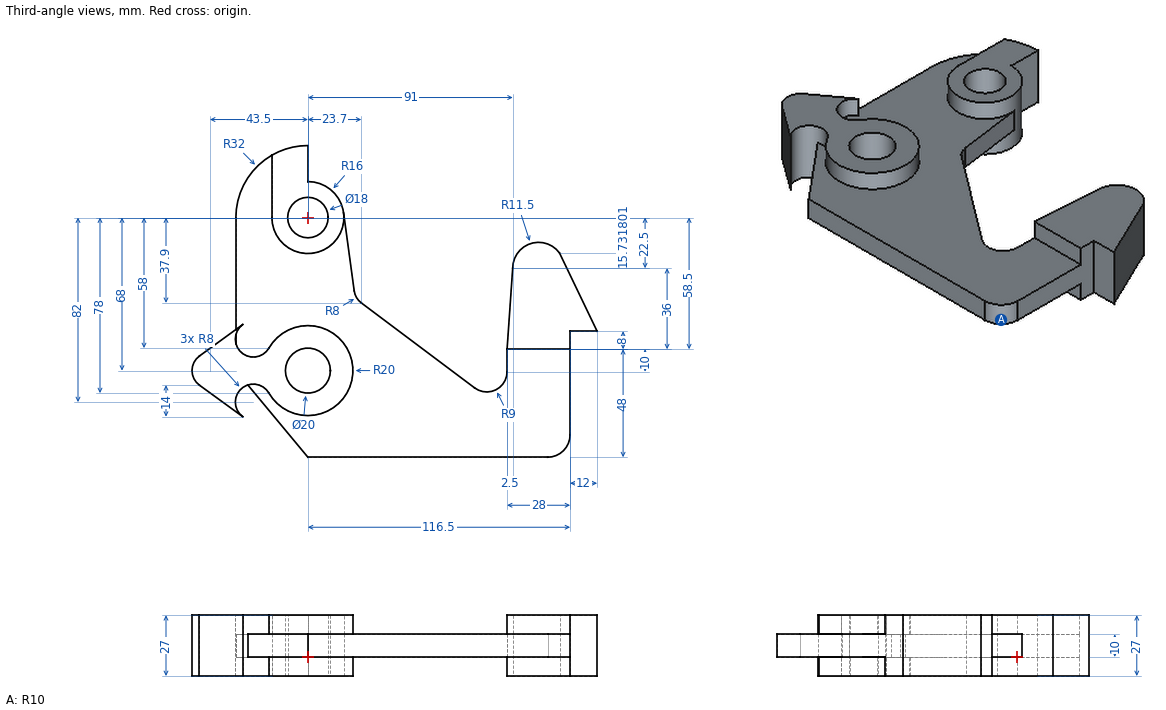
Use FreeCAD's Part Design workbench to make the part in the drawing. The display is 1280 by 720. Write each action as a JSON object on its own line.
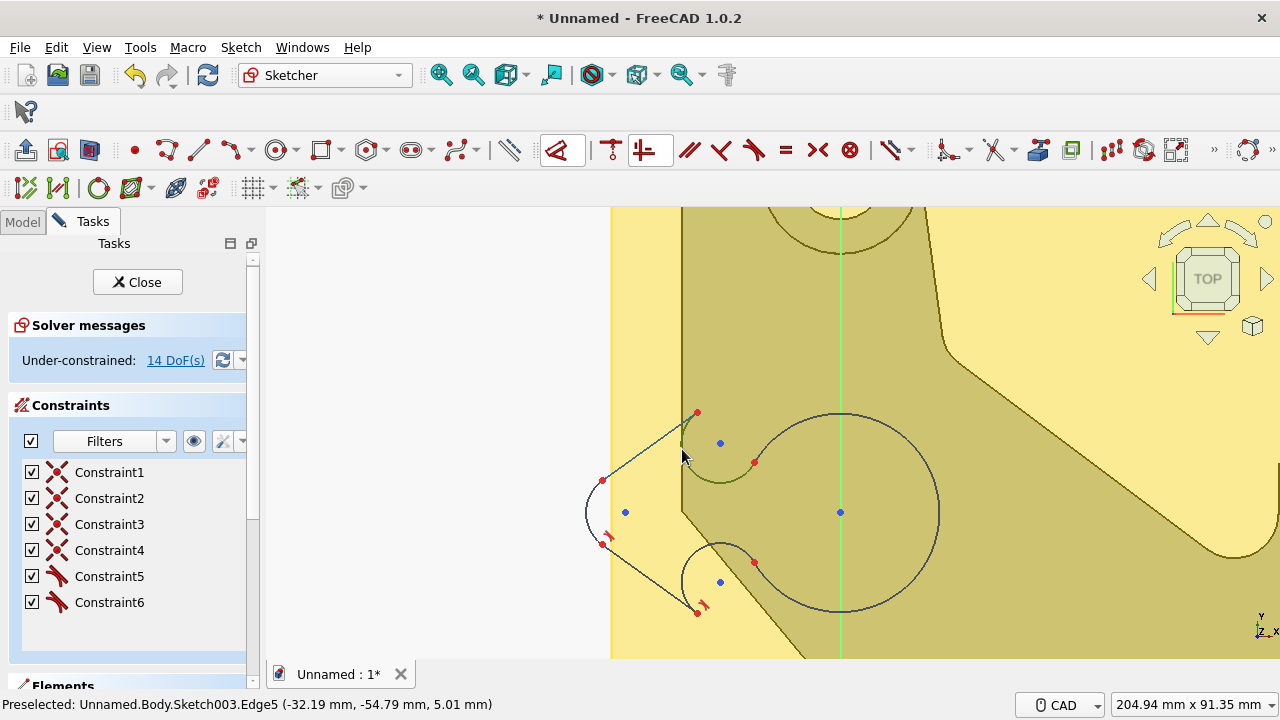
{"action": "key", "text": "t"}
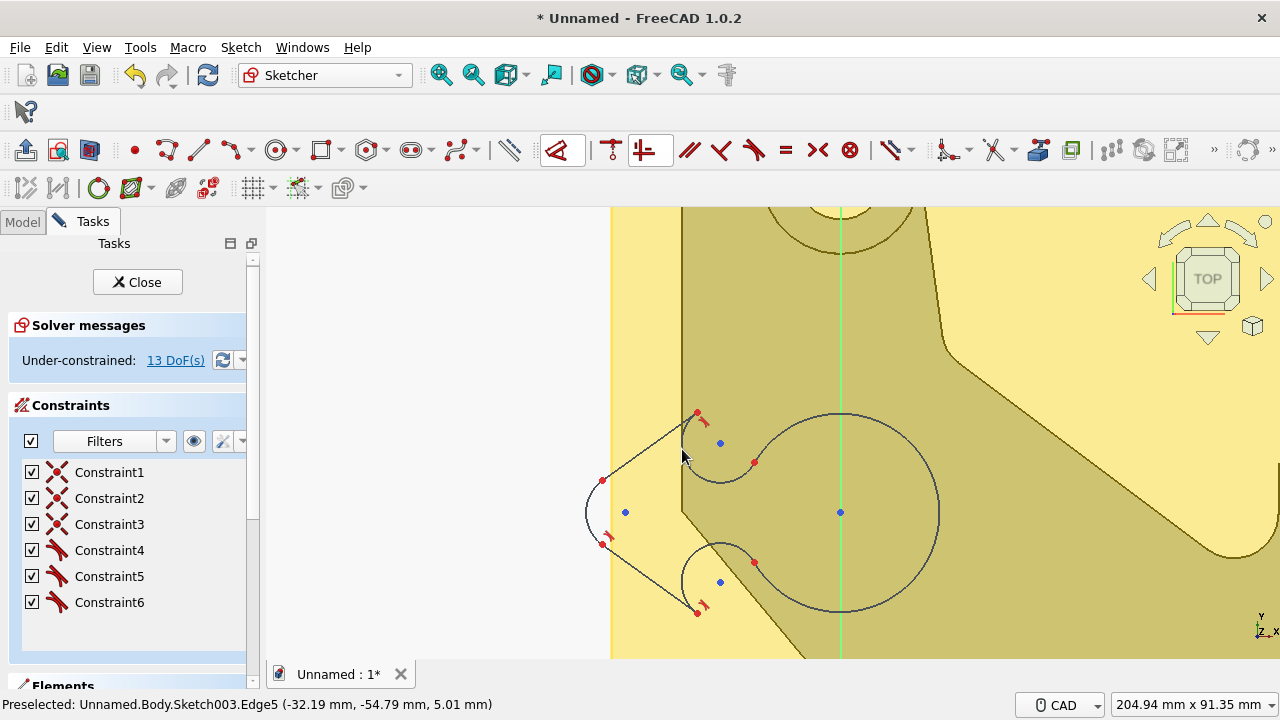
{"action": "left_click", "coordinate": [669, 433]}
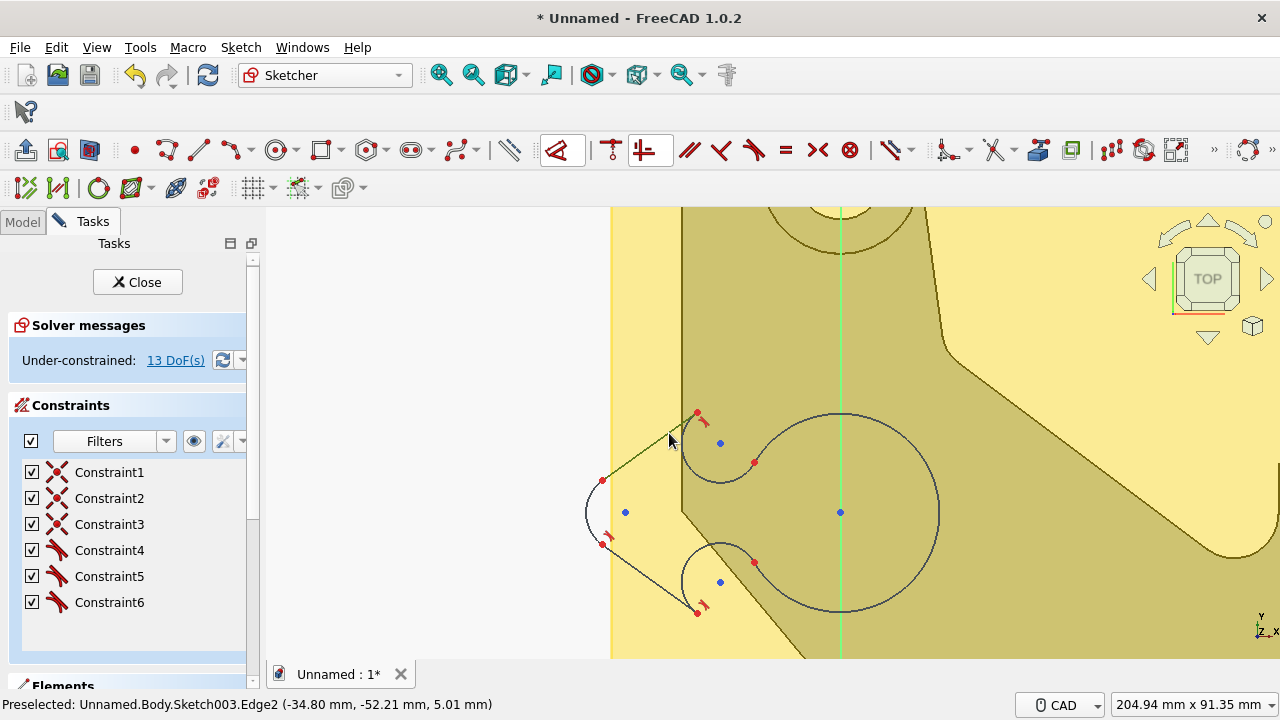
{"action": "left_click", "coordinate": [589, 498]}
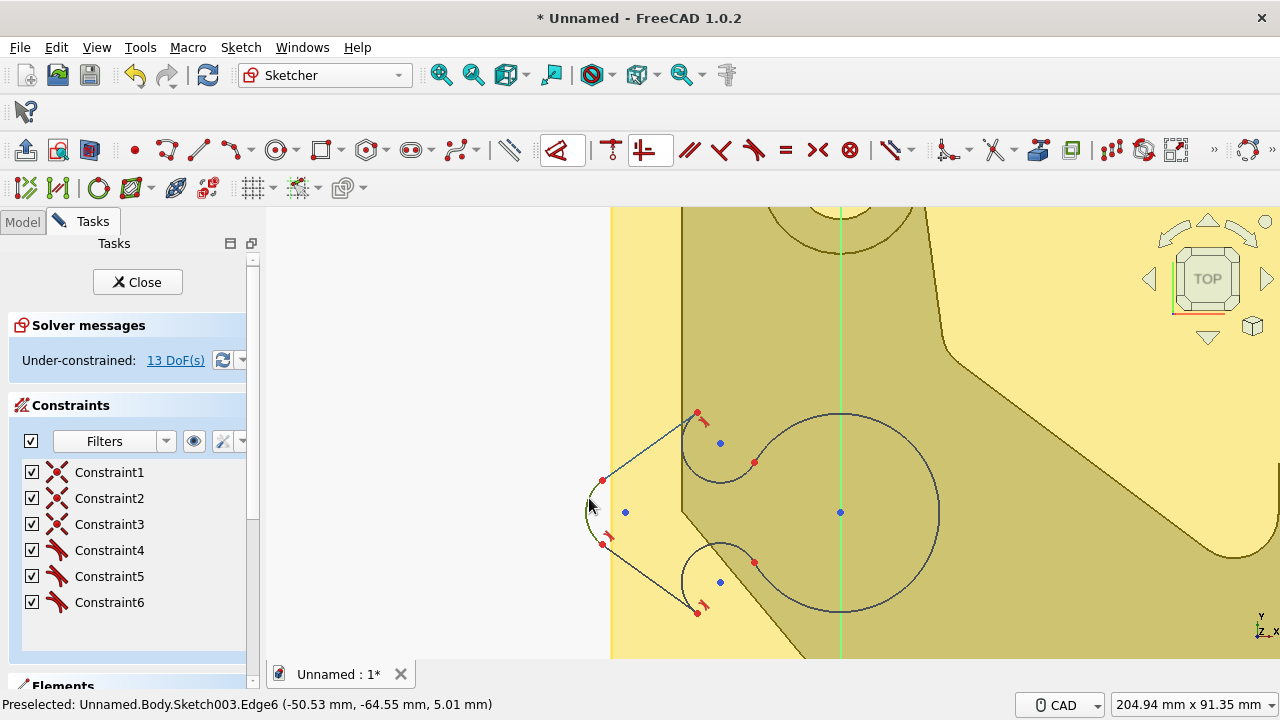
{"action": "left_click", "coordinate": [754, 150]}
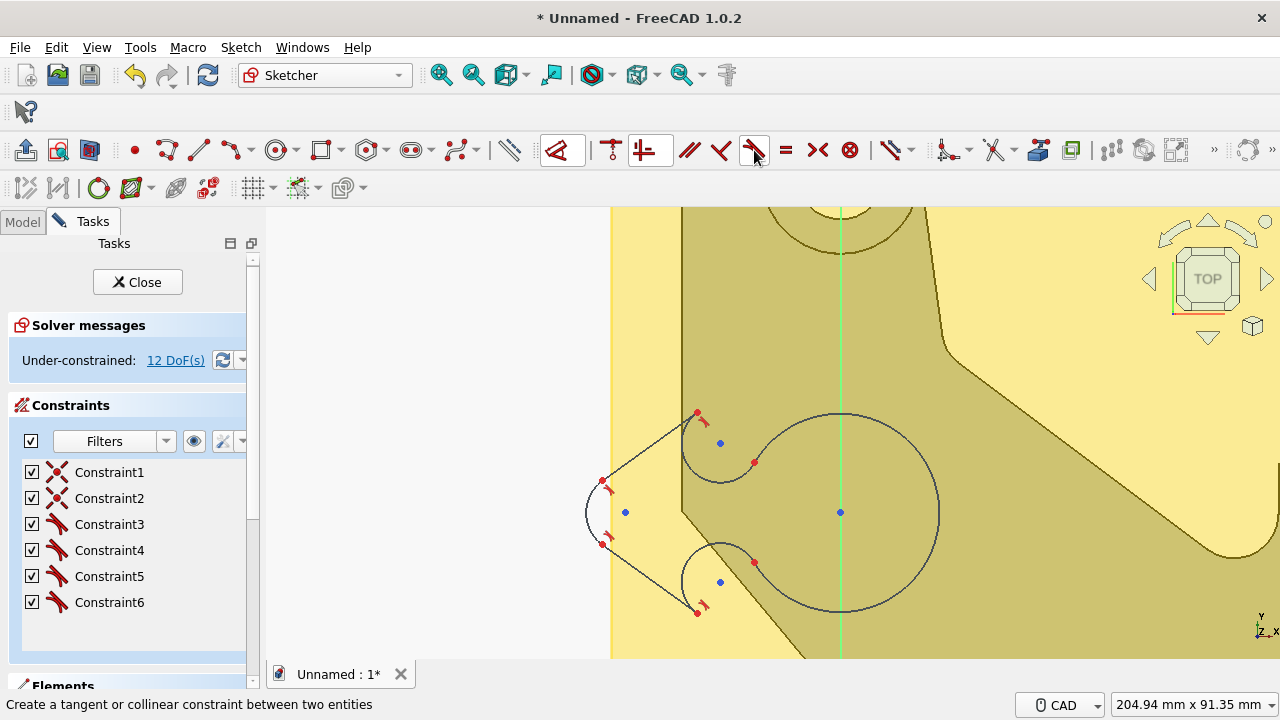
{"action": "left_click", "coordinate": [720, 543]}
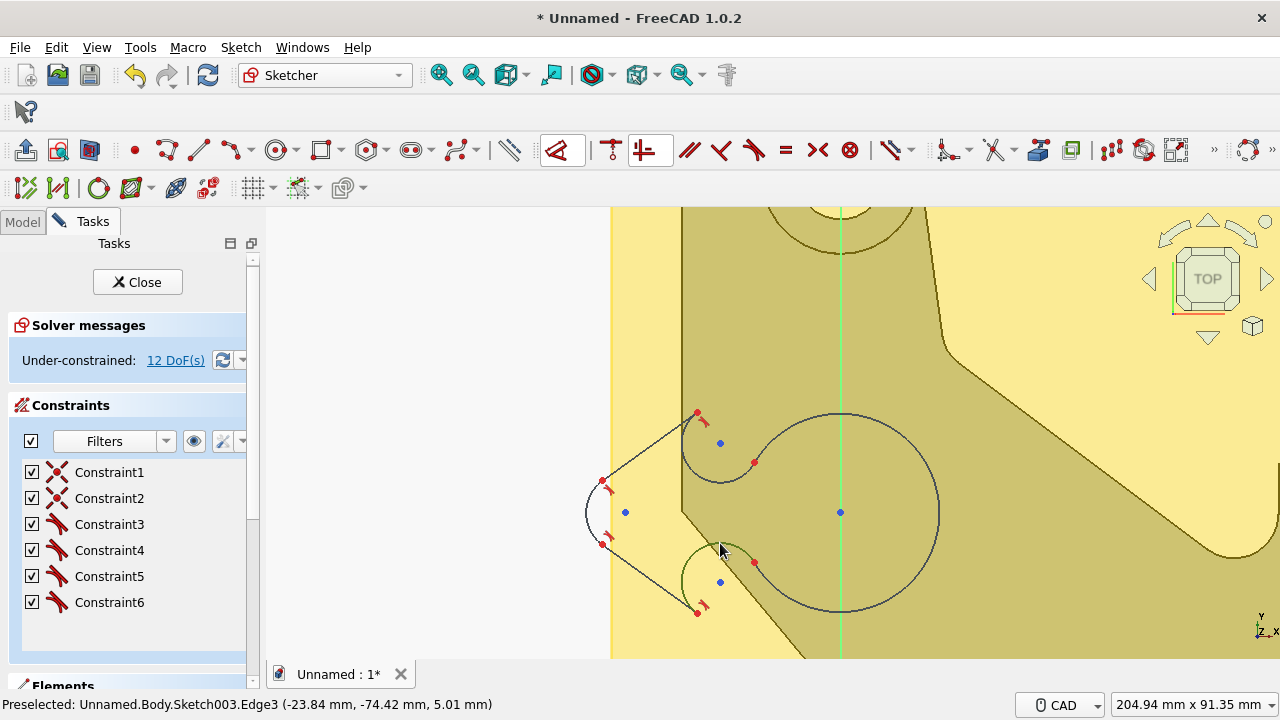
{"action": "left_click", "coordinate": [890, 599]}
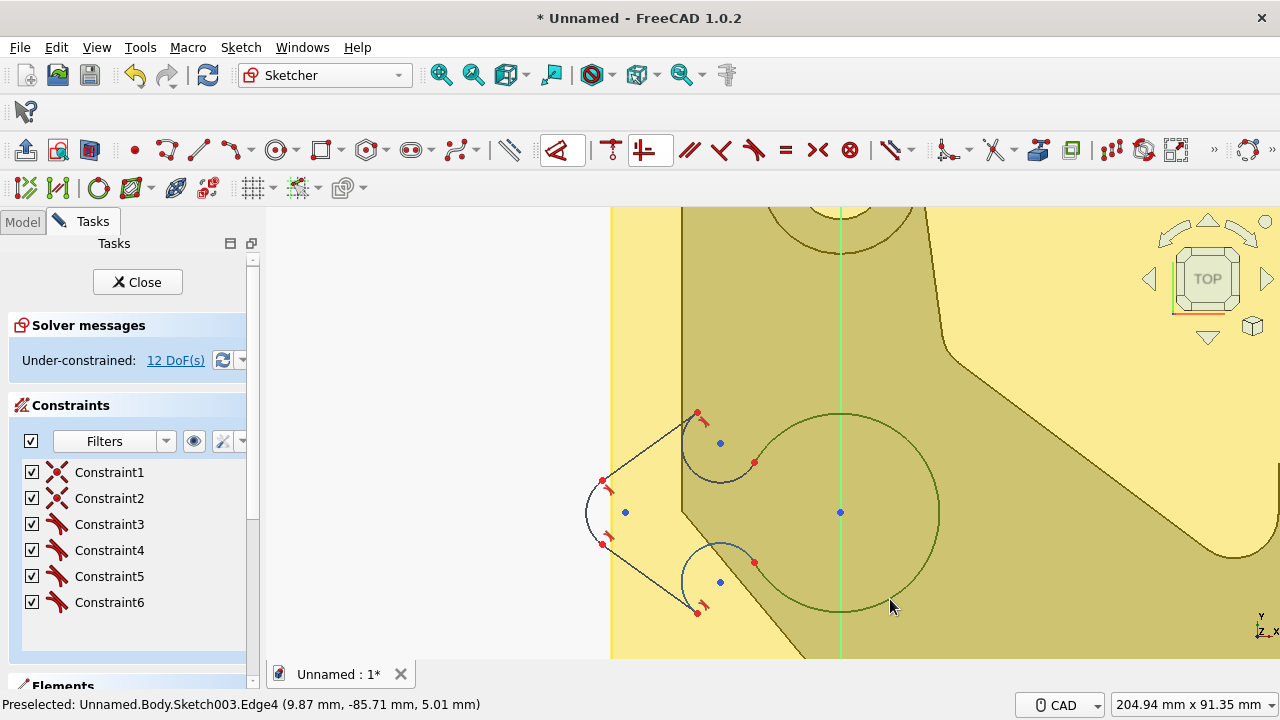
{"action": "key", "text": "t"}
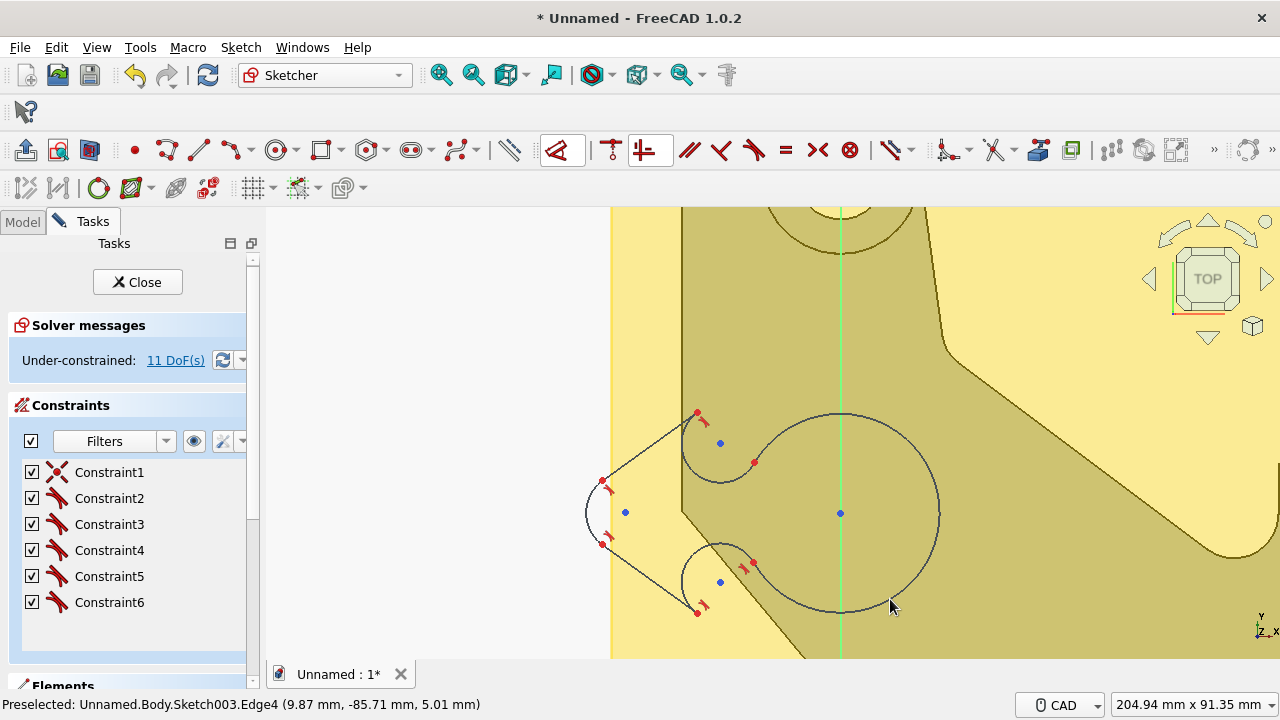
{"action": "left_click", "coordinate": [890, 600]}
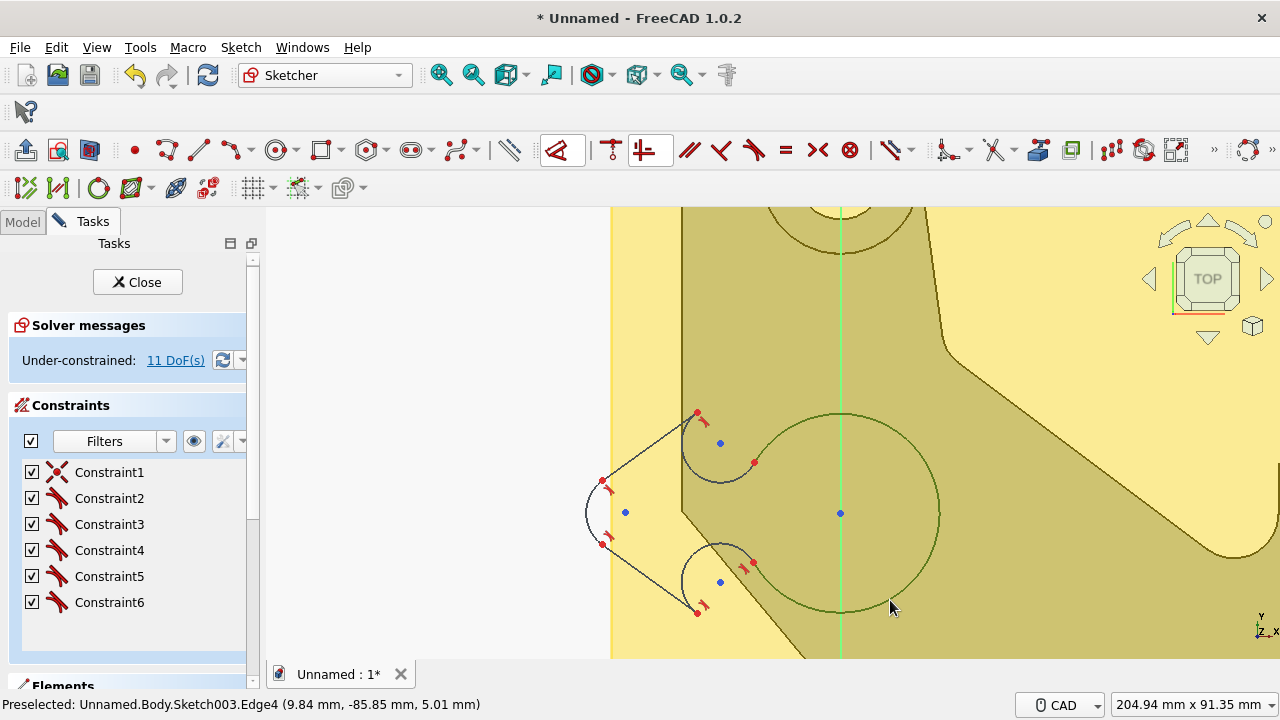
{"action": "left_click", "coordinate": [682, 449]}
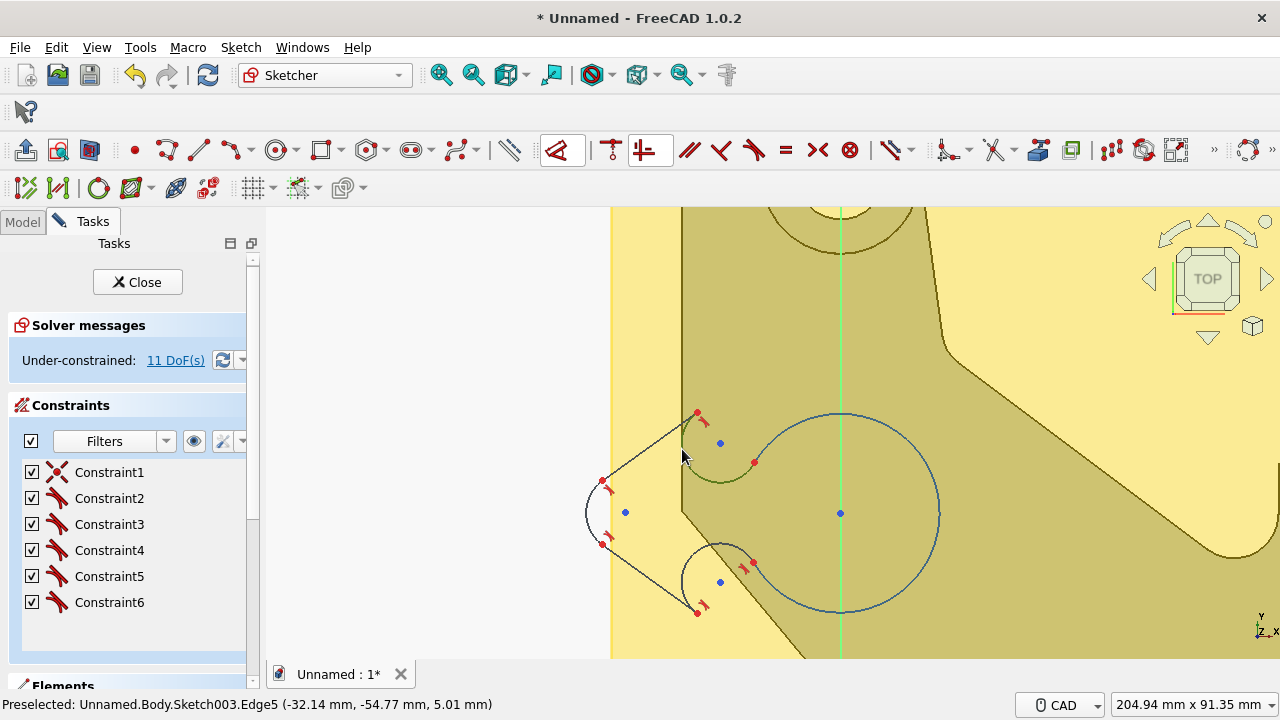
{"action": "key", "text": "t"}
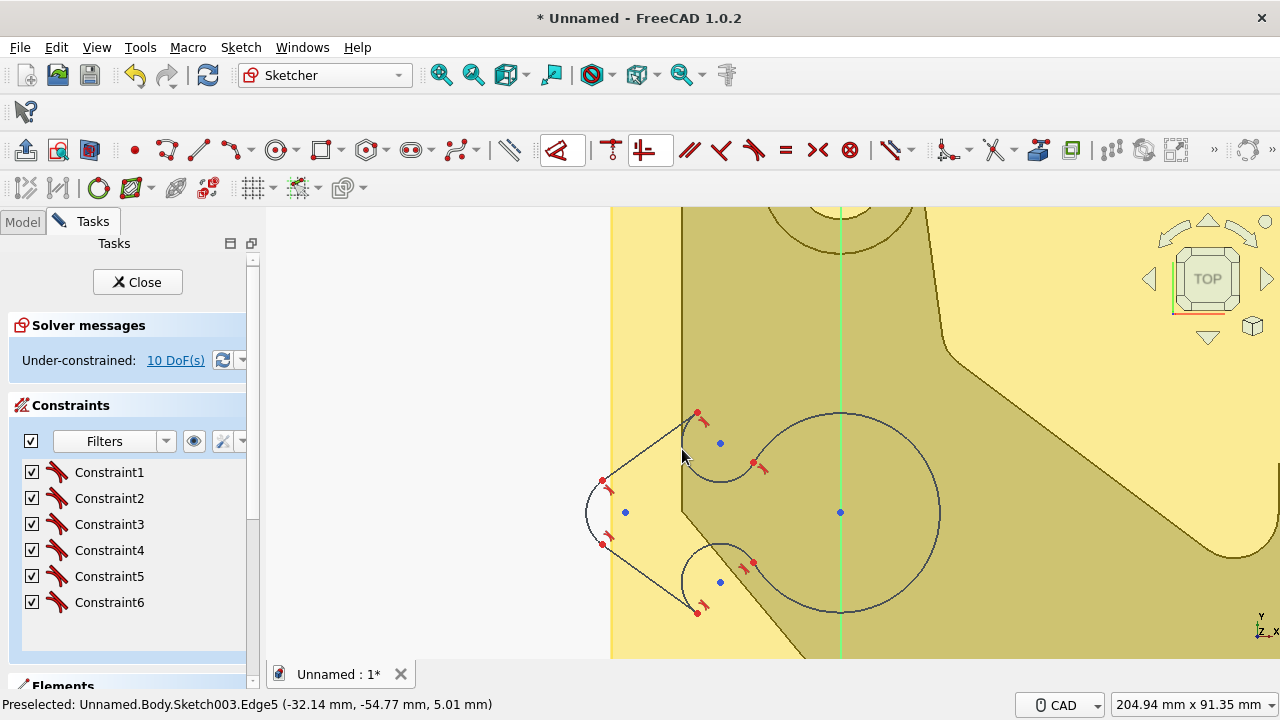
{"action": "left_click", "coordinate": [719, 544]}